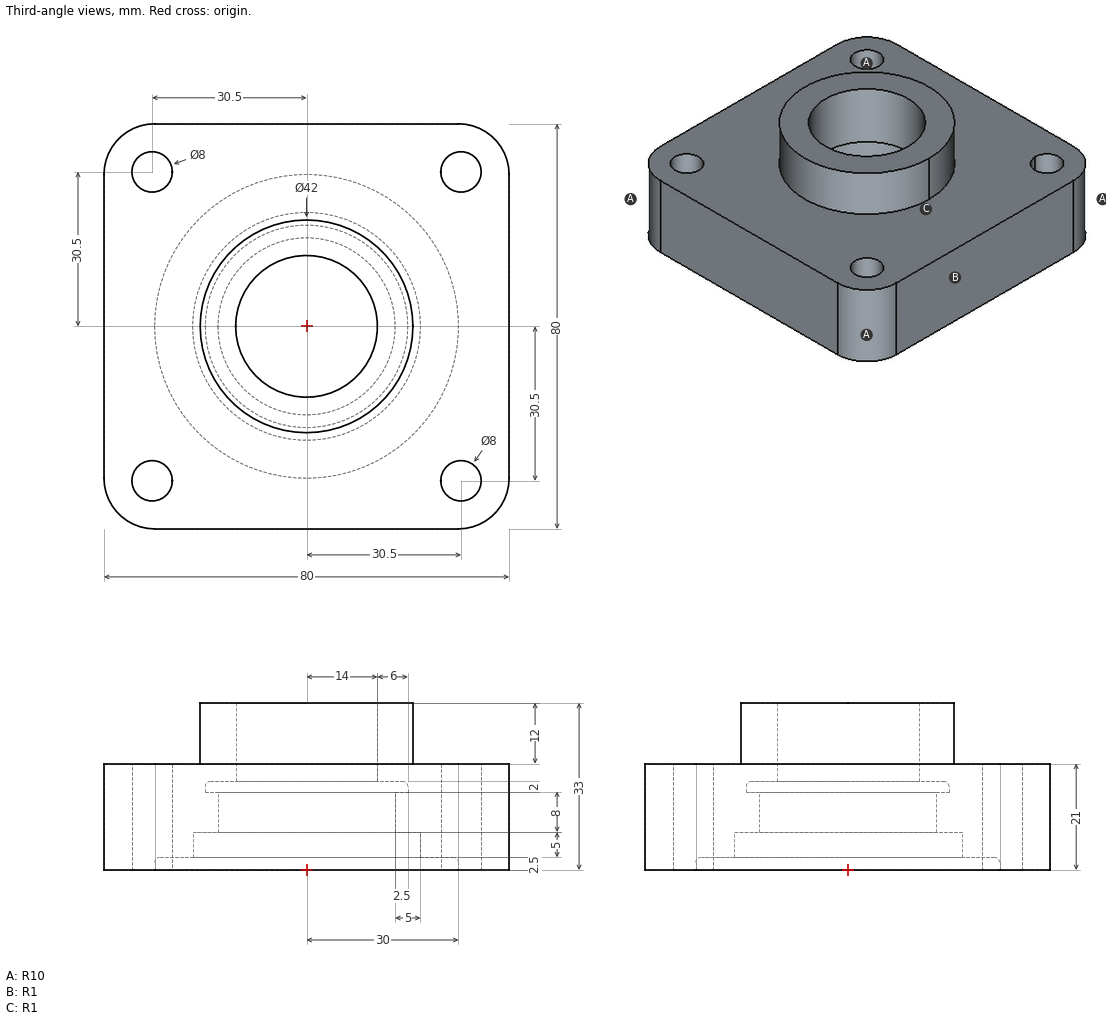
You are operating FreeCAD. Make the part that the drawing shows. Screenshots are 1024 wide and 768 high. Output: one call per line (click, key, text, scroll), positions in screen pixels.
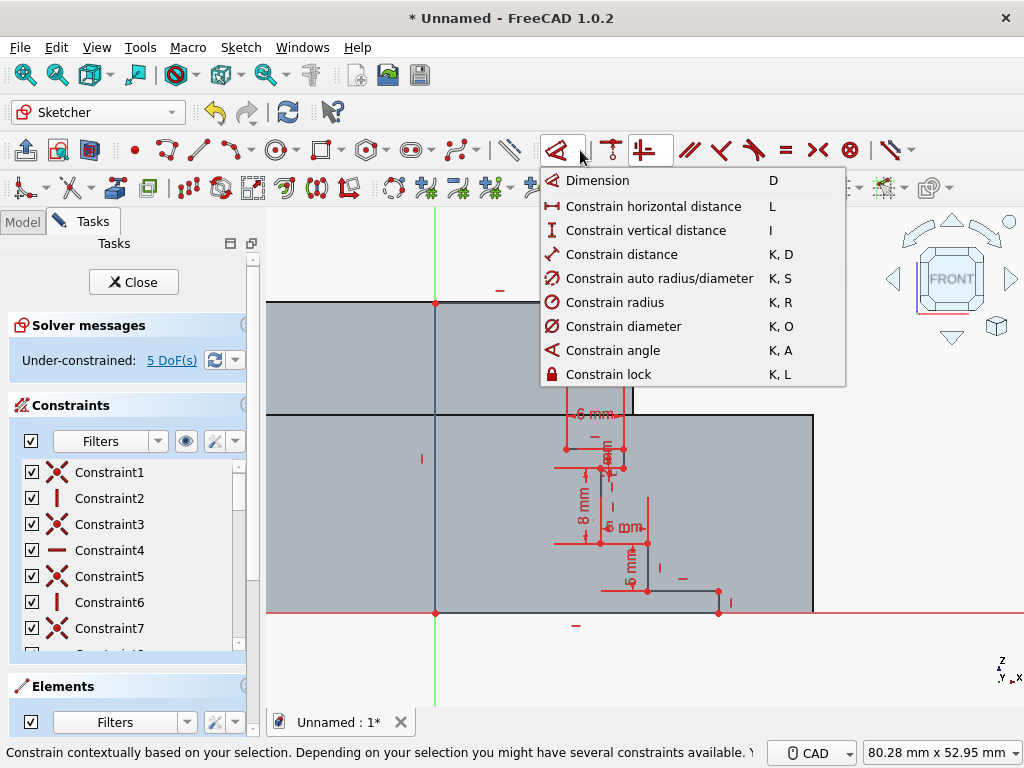
click(693, 230)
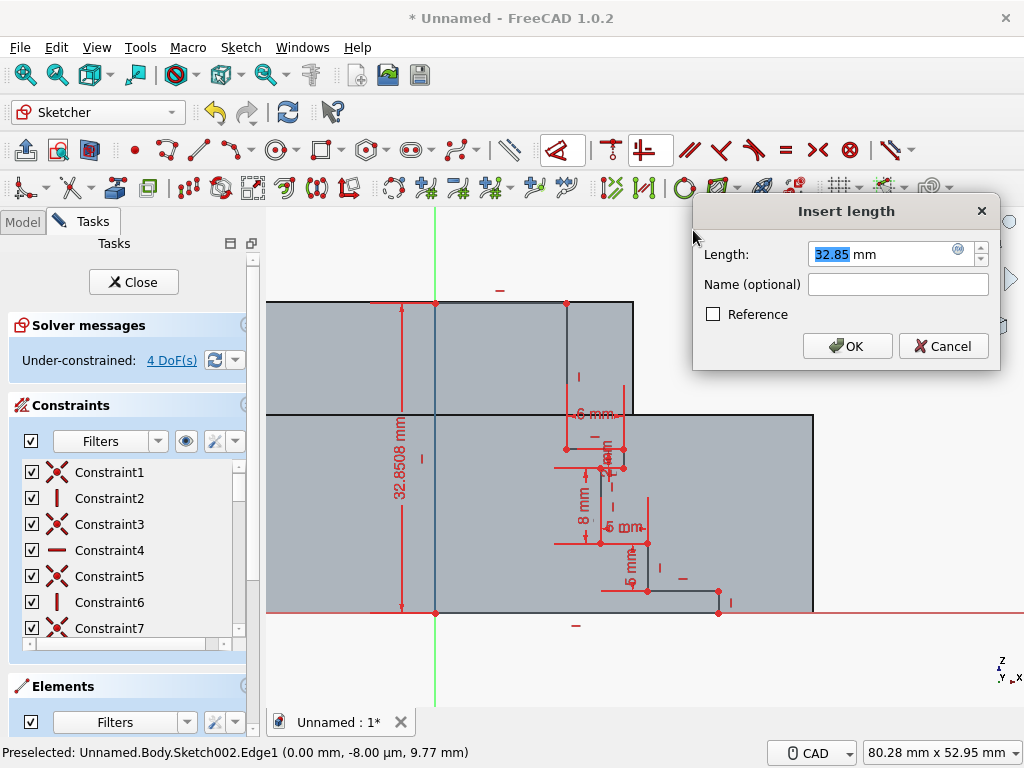
text(33)
key(Return)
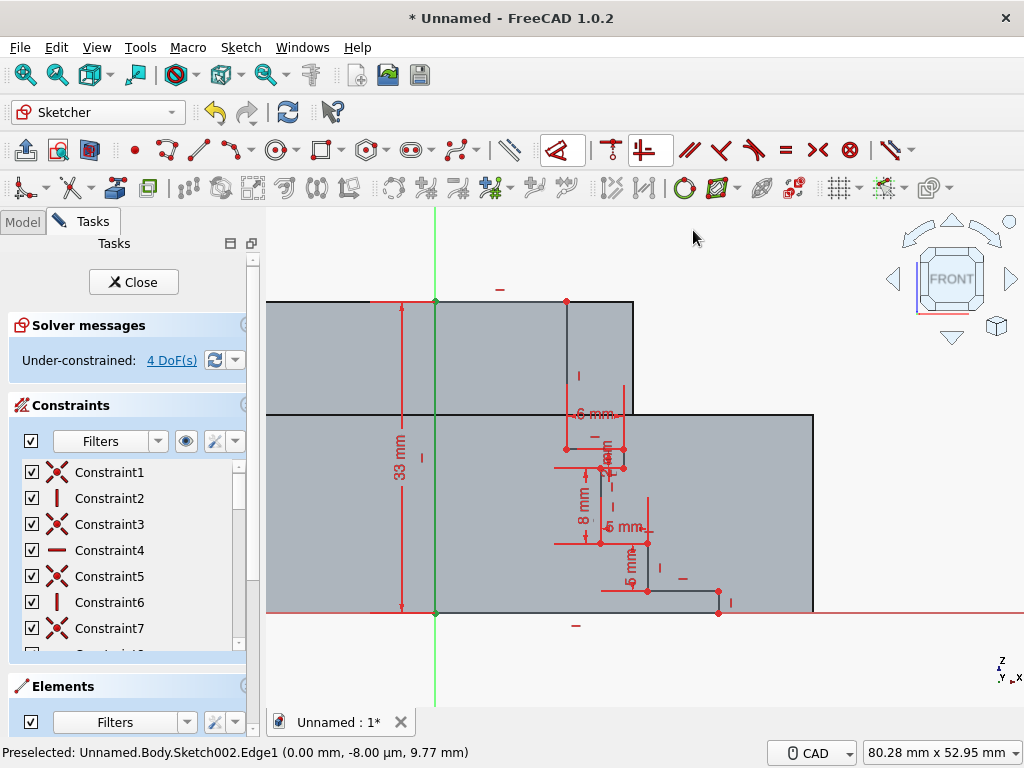
click(475, 302)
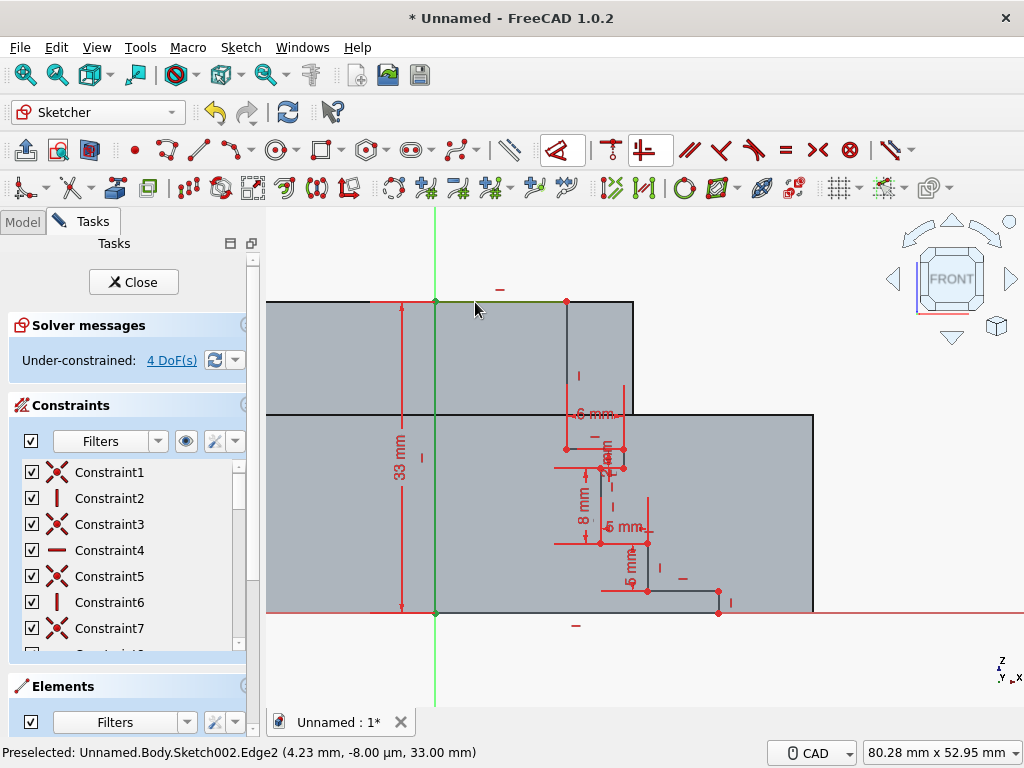
click(580, 150)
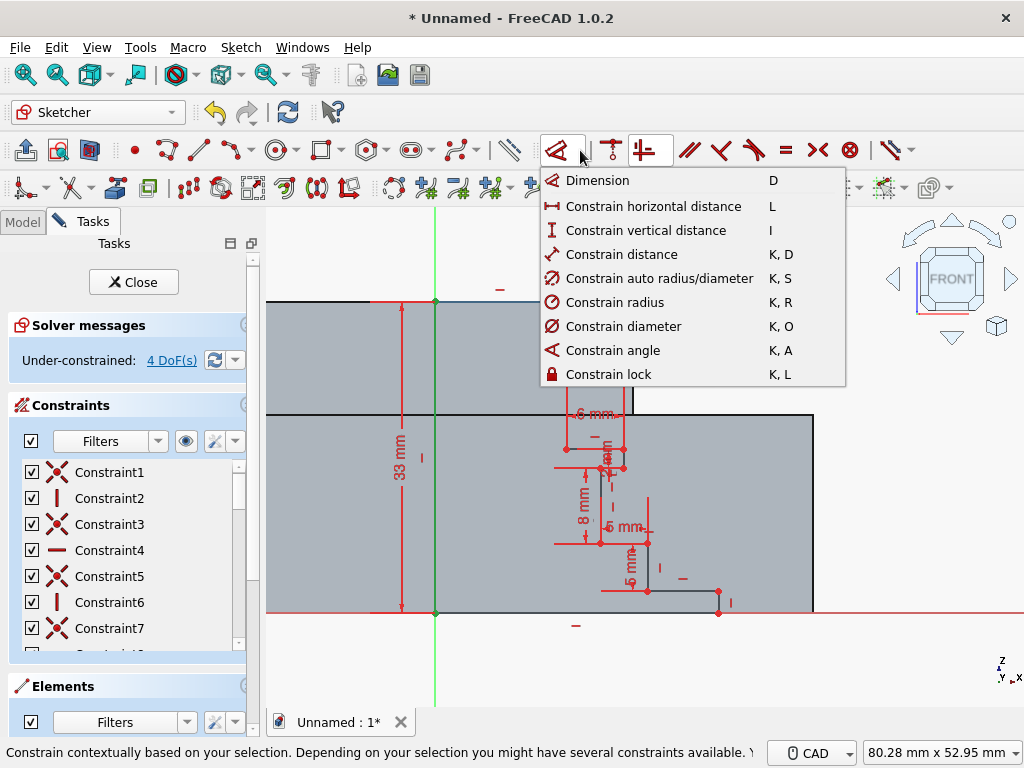
click(693, 206)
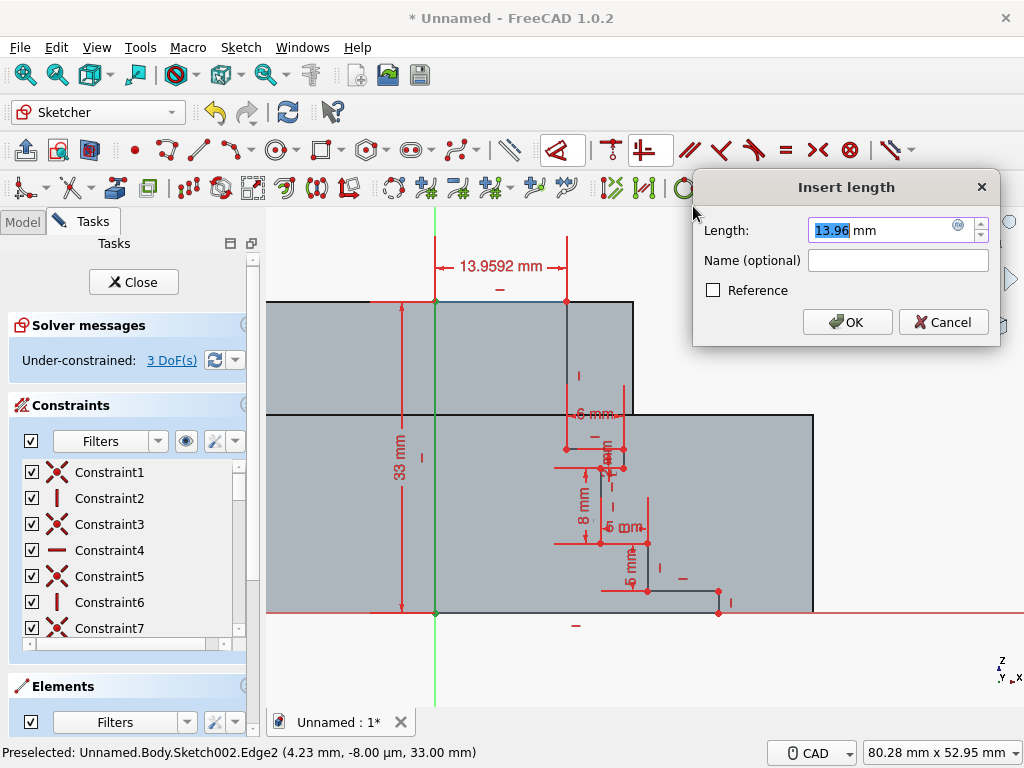
text(14)
key(Return)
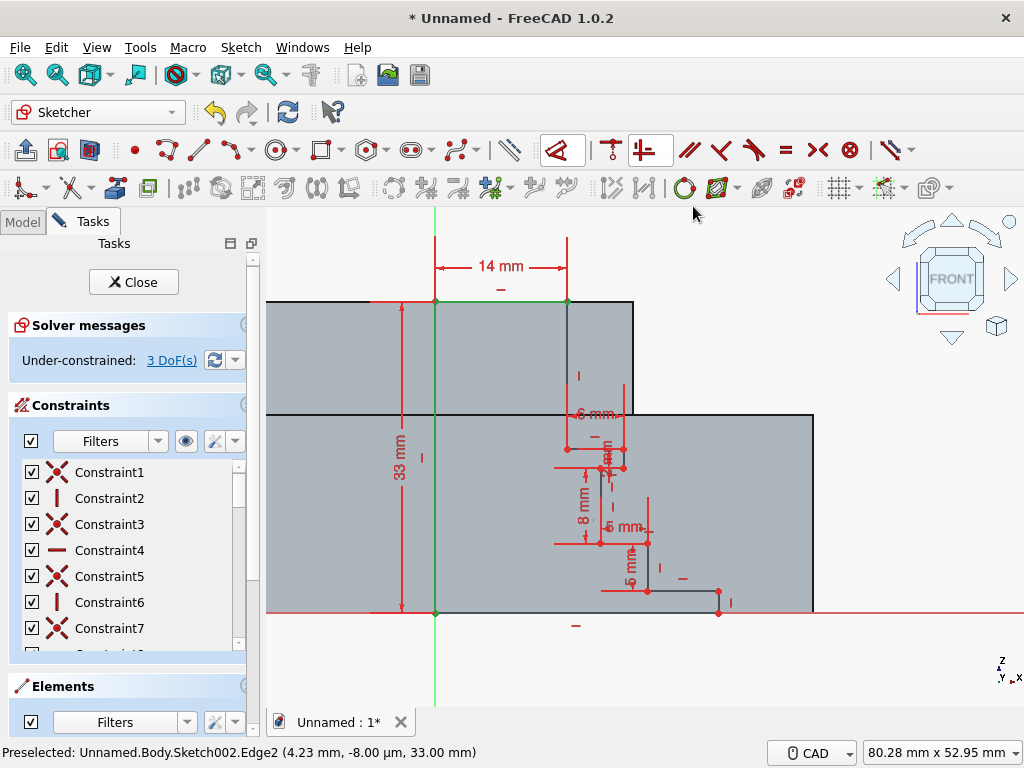
click(634, 613)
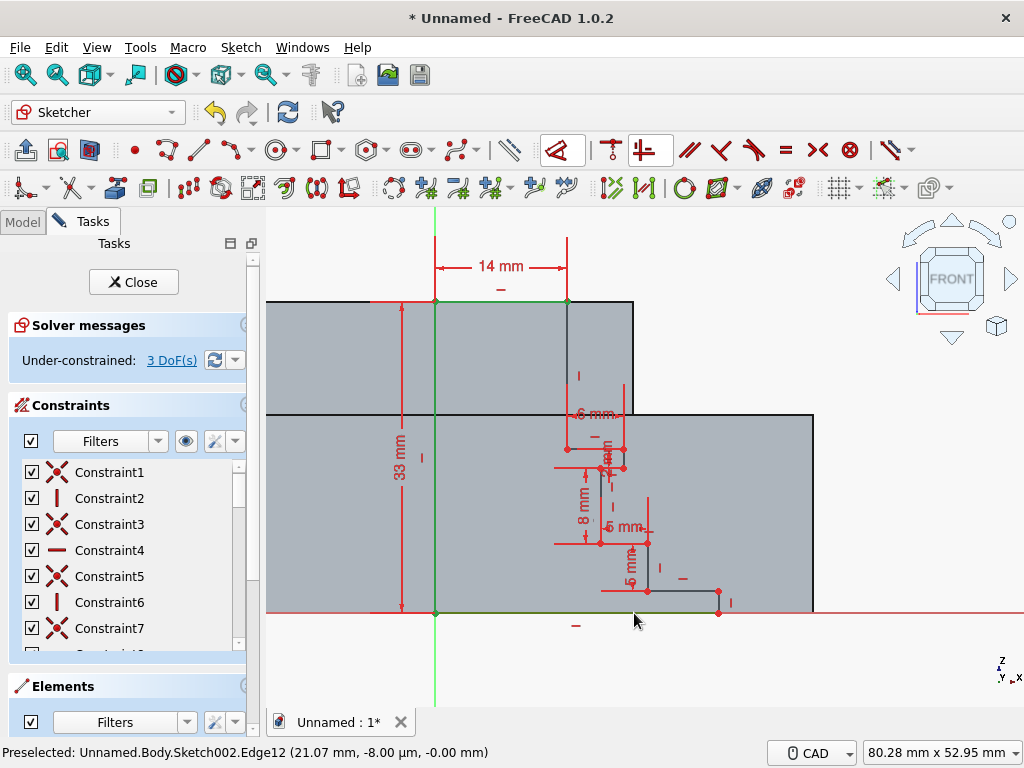
key(l)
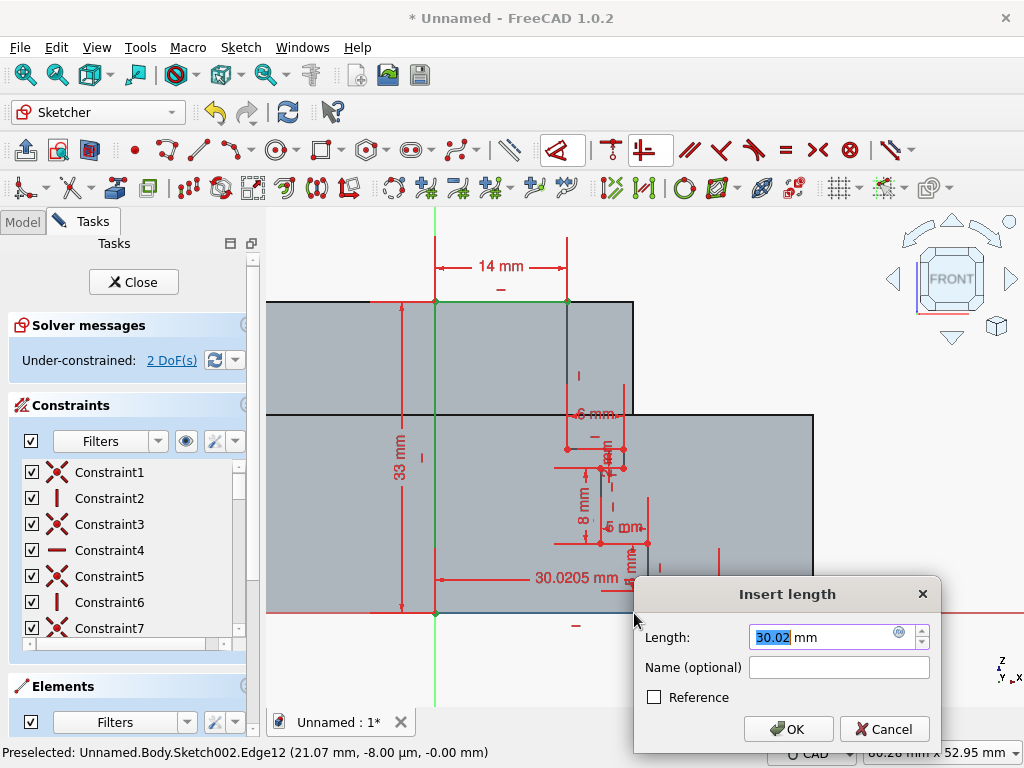
text(30)
key(Return)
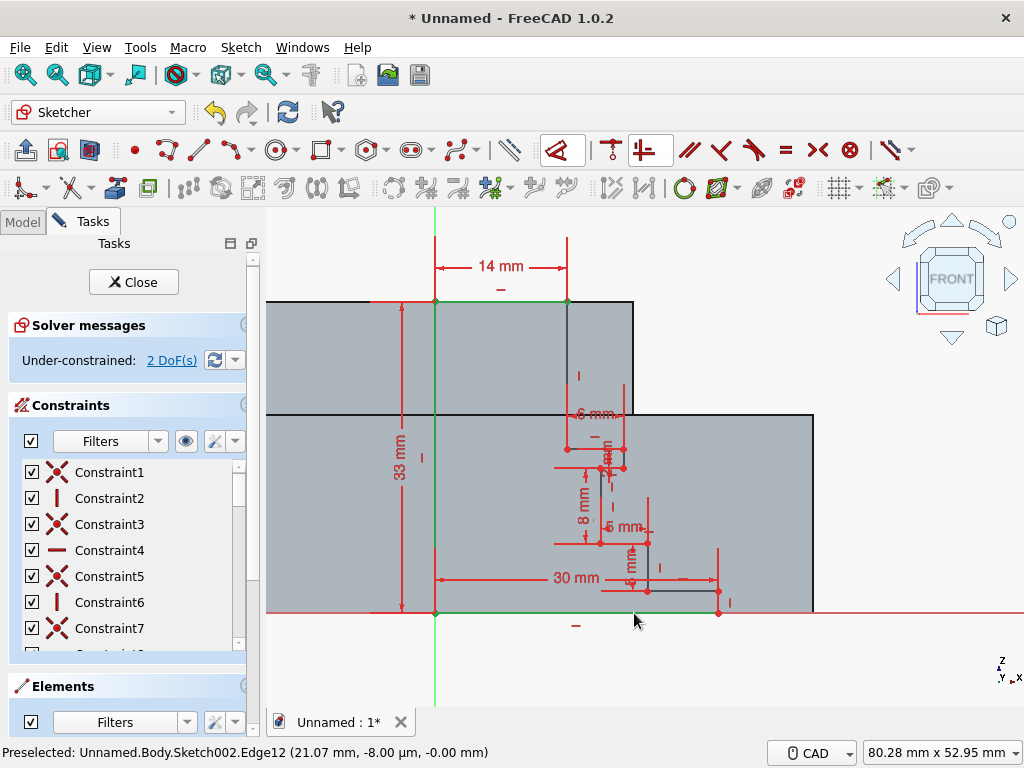
scroll(615, 468, up, 3)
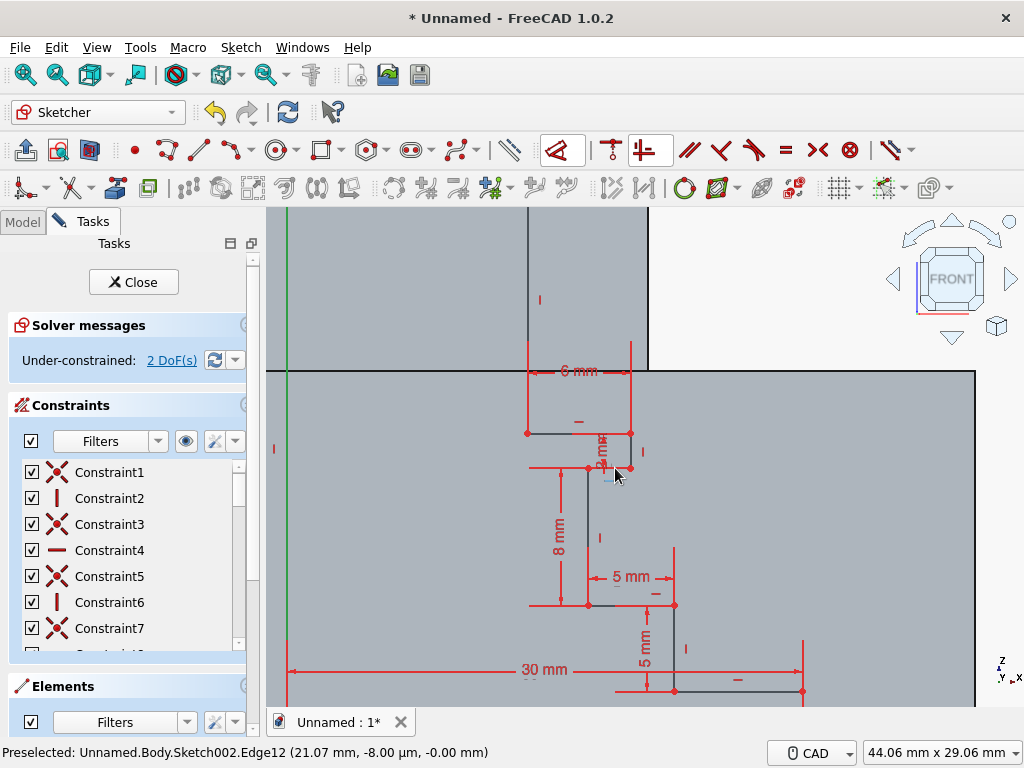
click(614, 468)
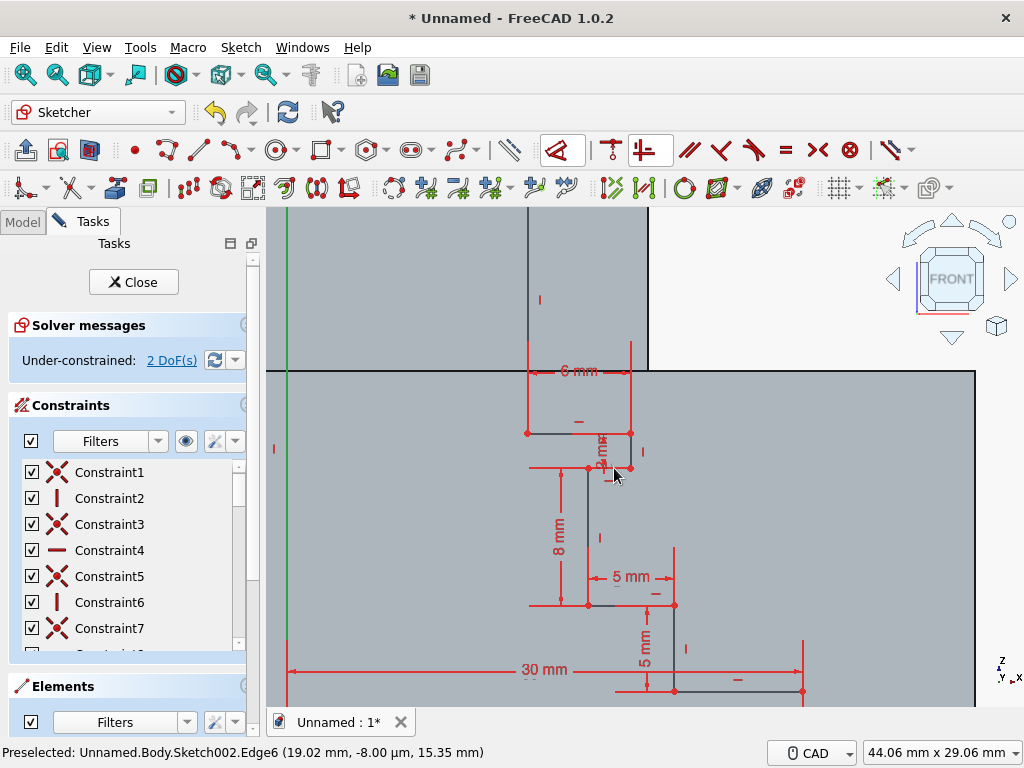
click(580, 150)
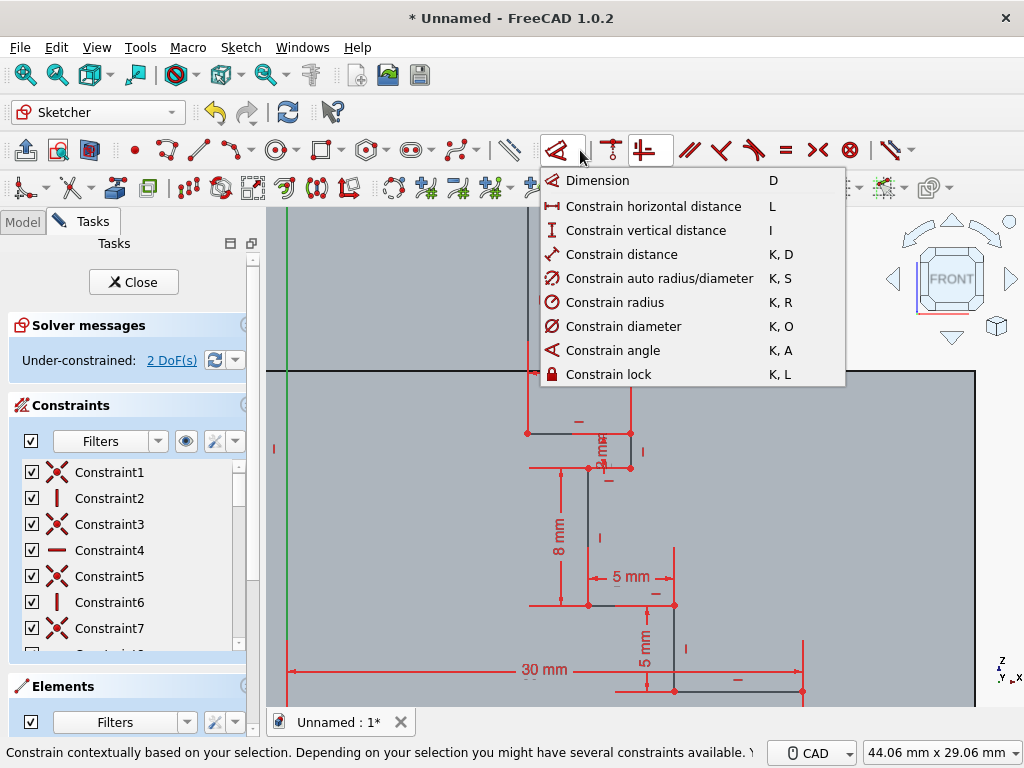
click(693, 206)